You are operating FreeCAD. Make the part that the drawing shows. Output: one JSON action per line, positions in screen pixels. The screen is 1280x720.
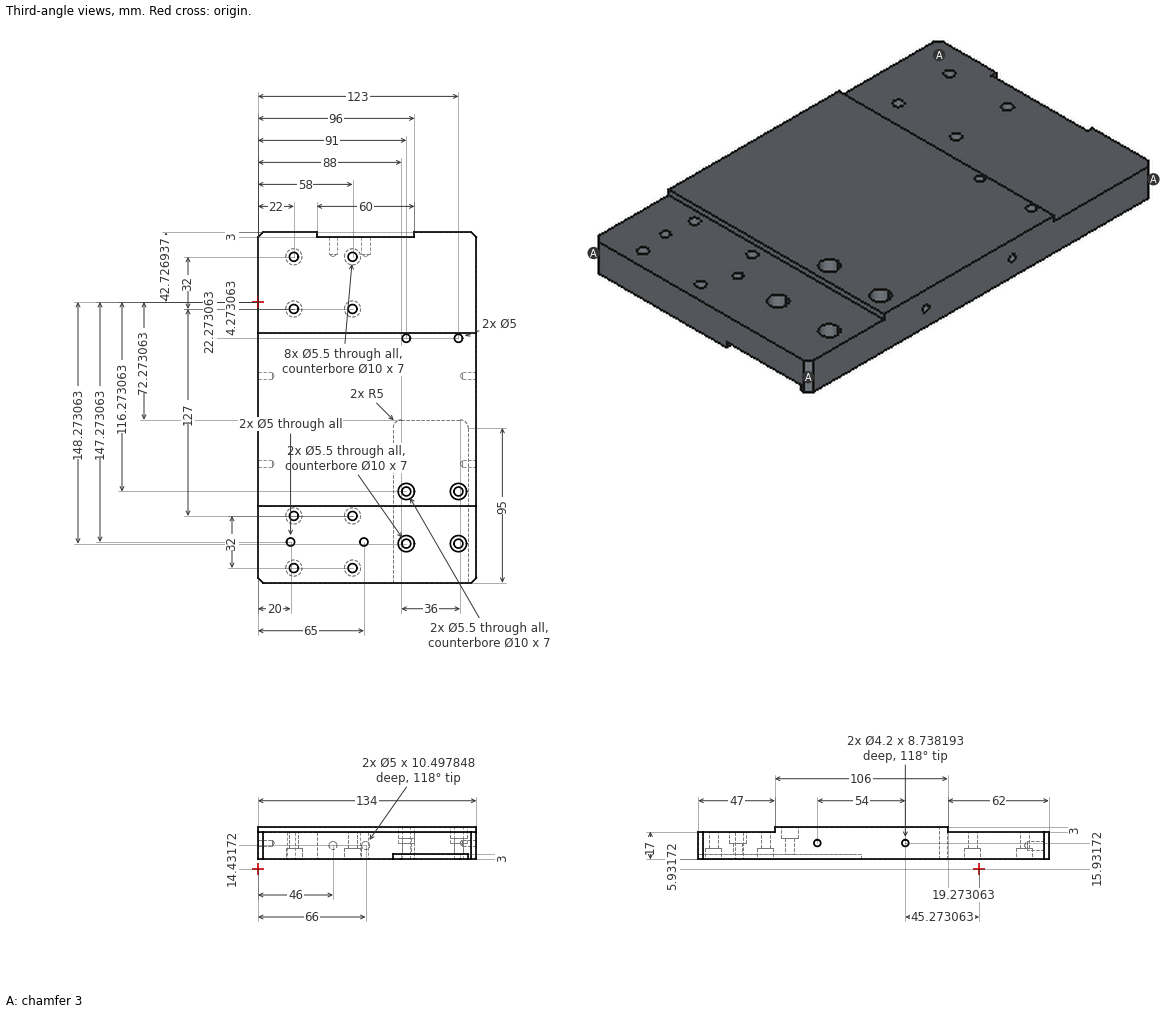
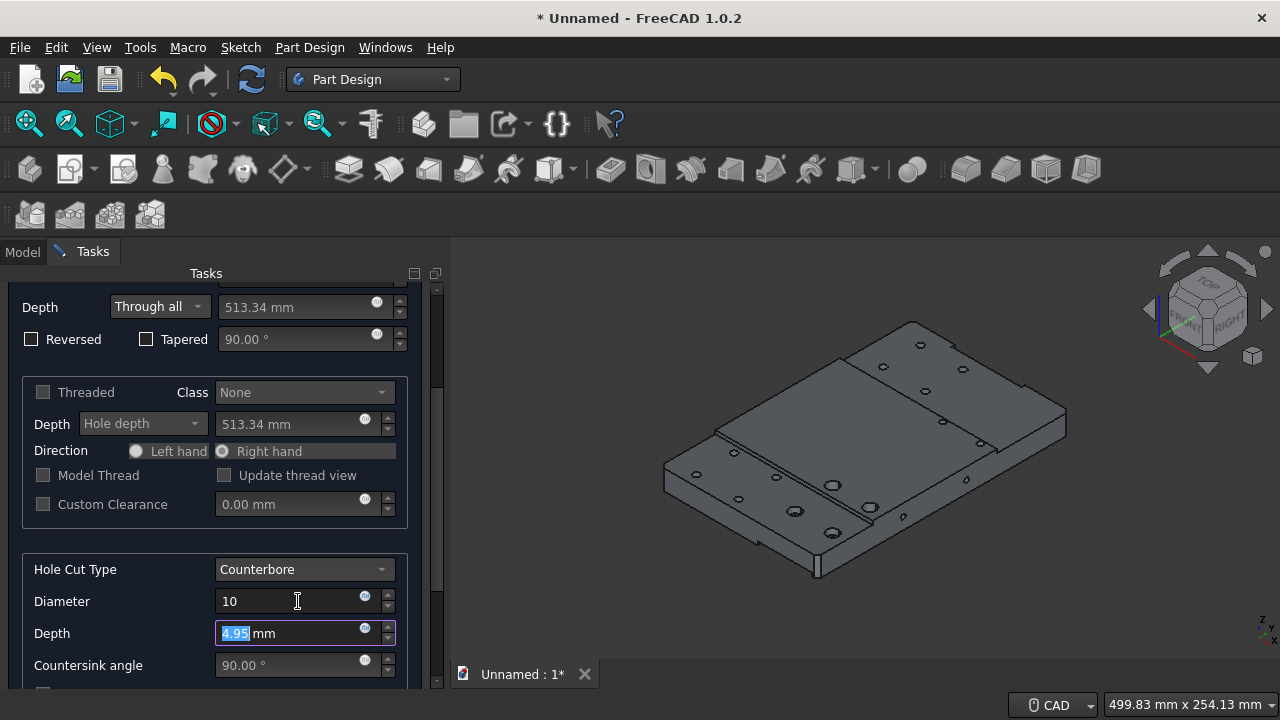
{"action": "type", "text": "7"}
{"action": "key", "text": "Tab"}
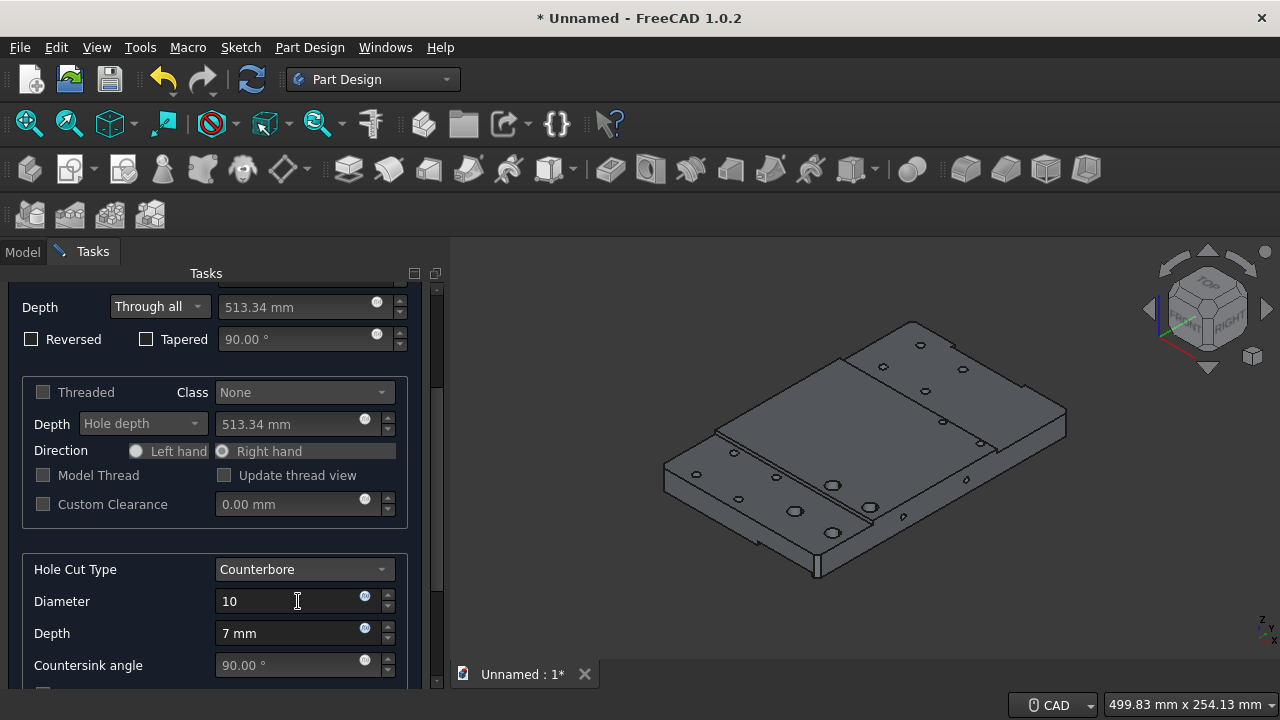
{"action": "scroll", "coordinate": [437, 486], "scroll_direction": "up", "scroll_amount": 4}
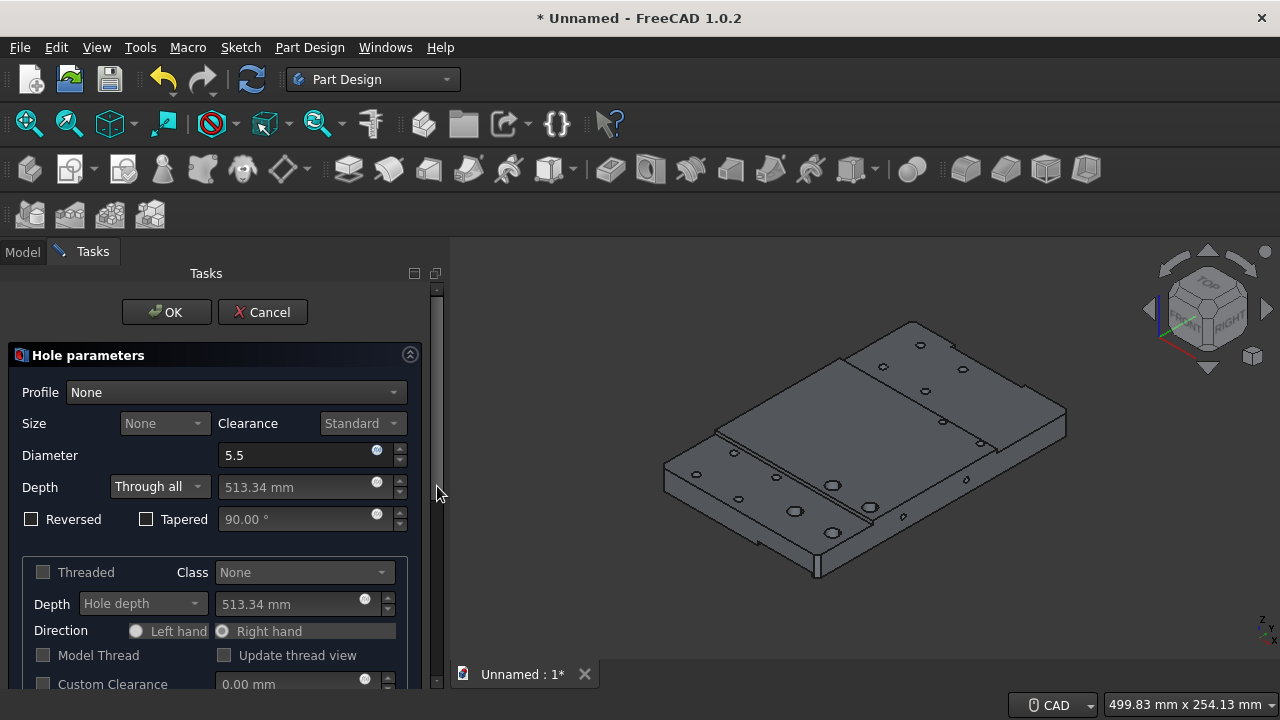
{"action": "left_click", "coordinate": [167, 312]}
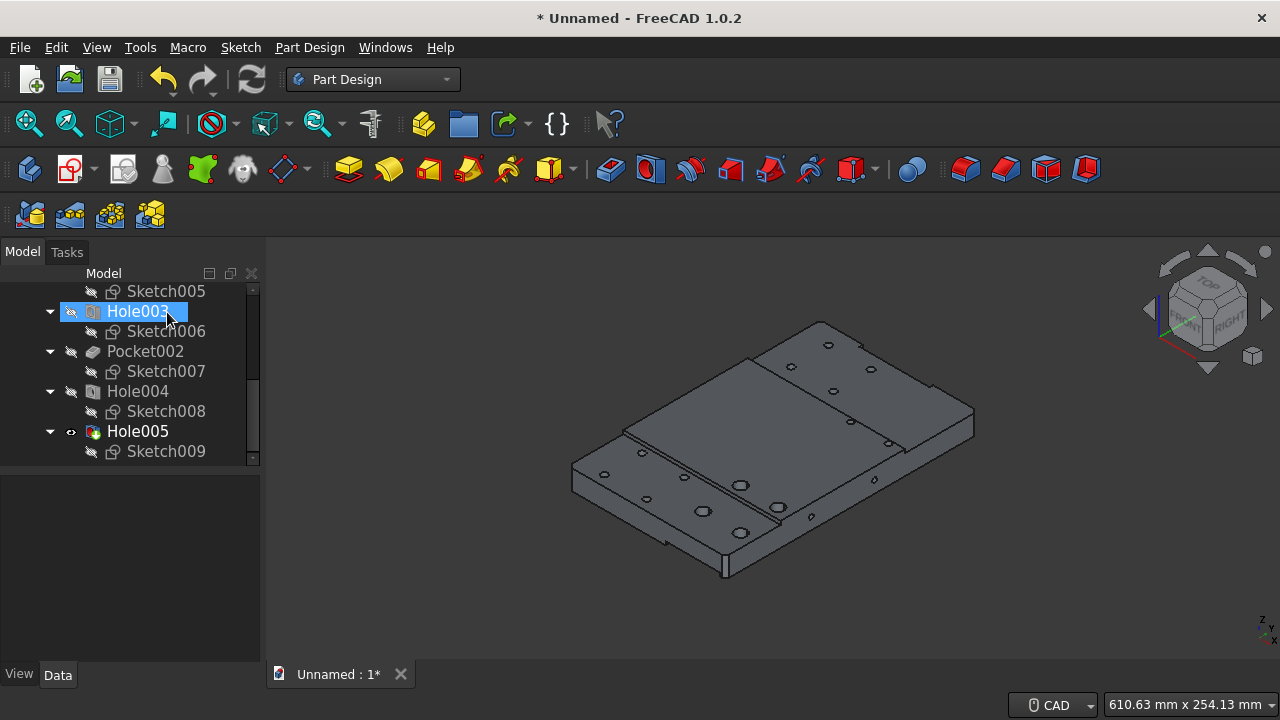
{"action": "left_click", "coordinate": [908, 412]}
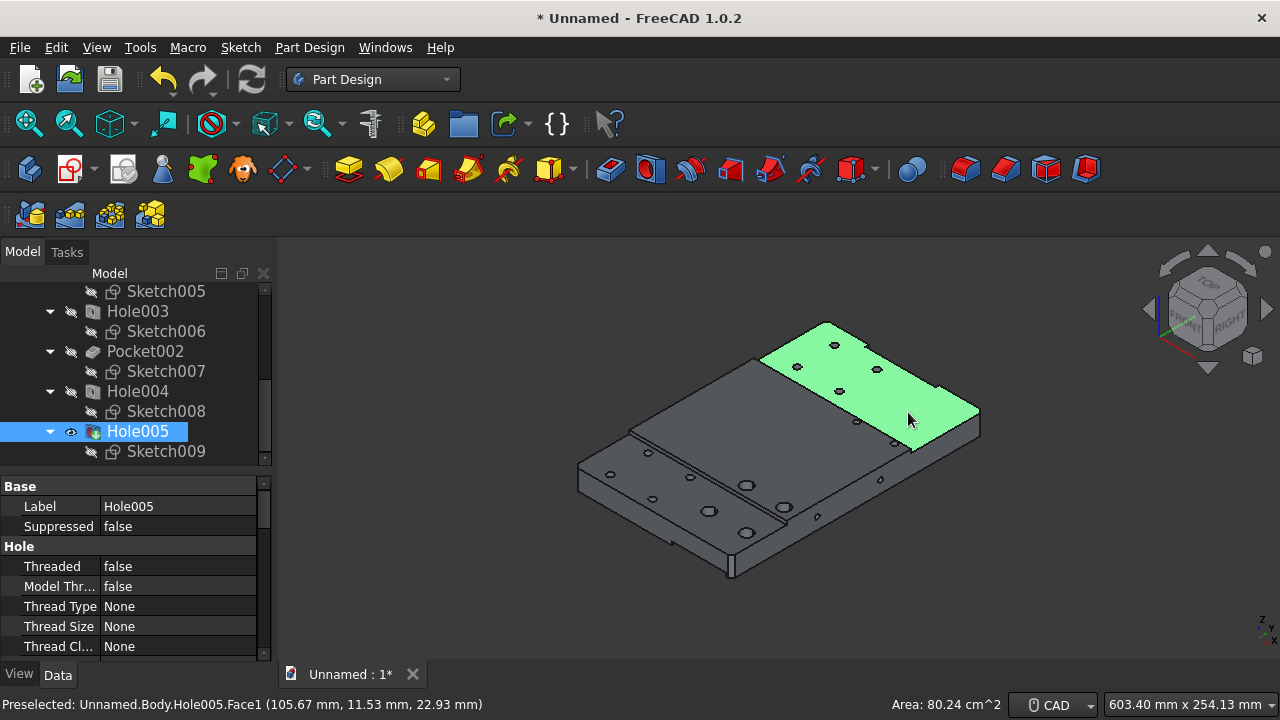
{"action": "left_click", "coordinate": [70, 170]}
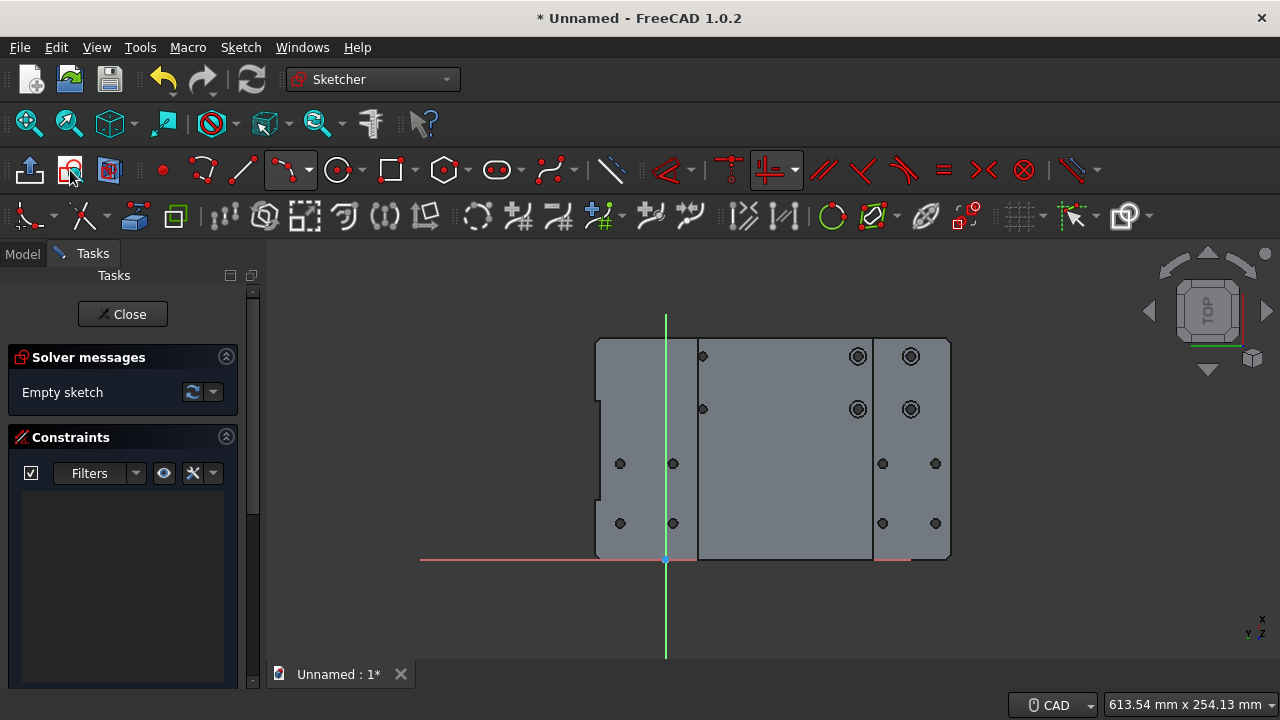
{"action": "scroll", "coordinate": [998, 507], "scroll_direction": "up", "scroll_amount": 6}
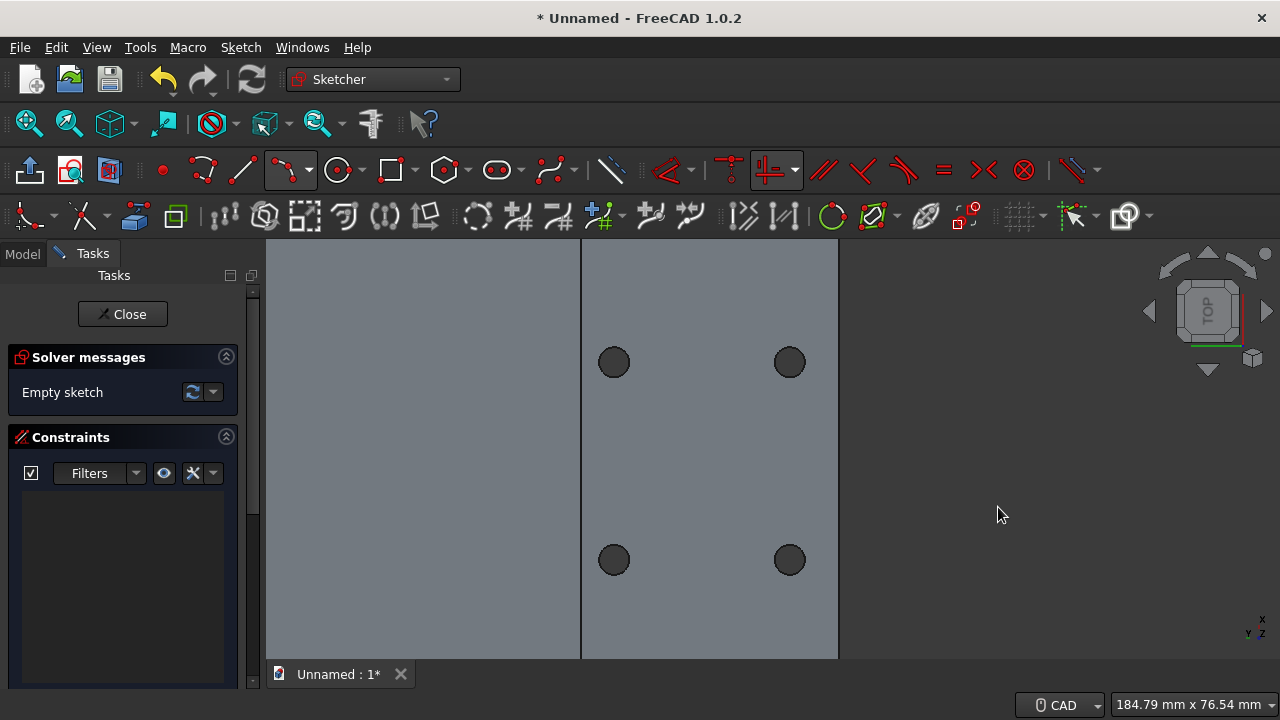
{"action": "left_click", "coordinate": [338, 170]}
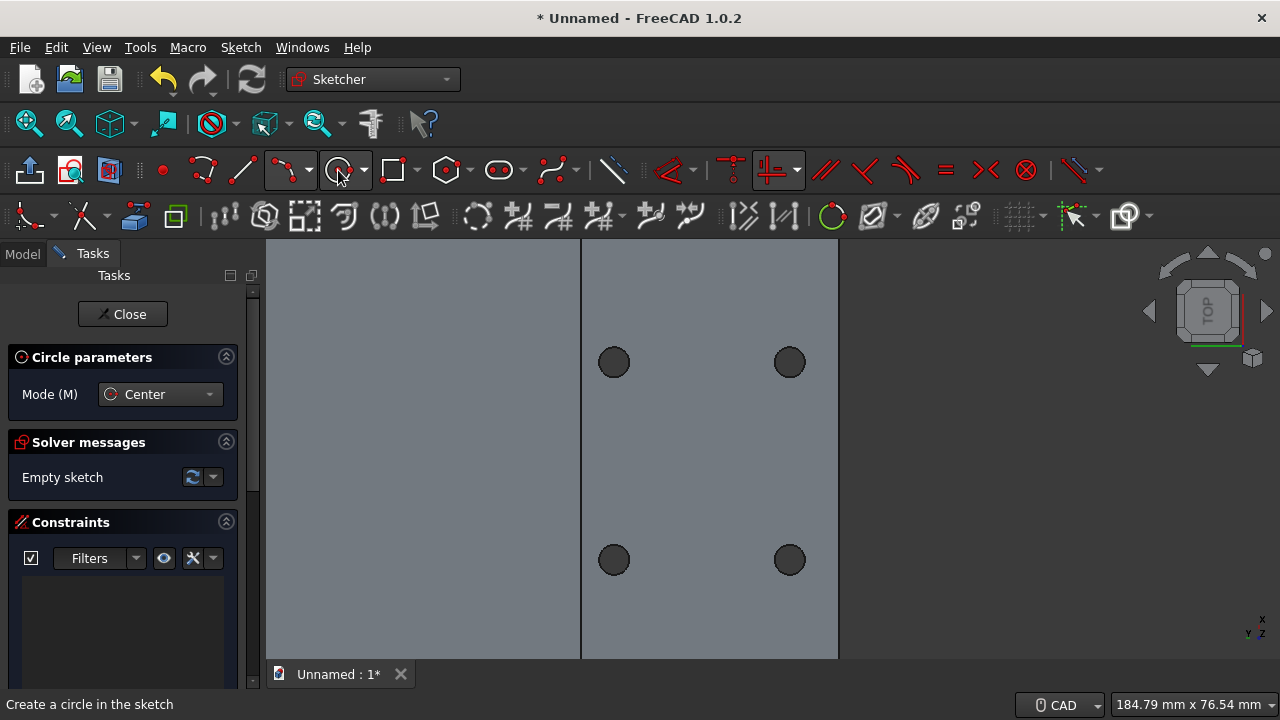
{"action": "scroll", "coordinate": [702, 571], "scroll_direction": "up", "scroll_amount": 3}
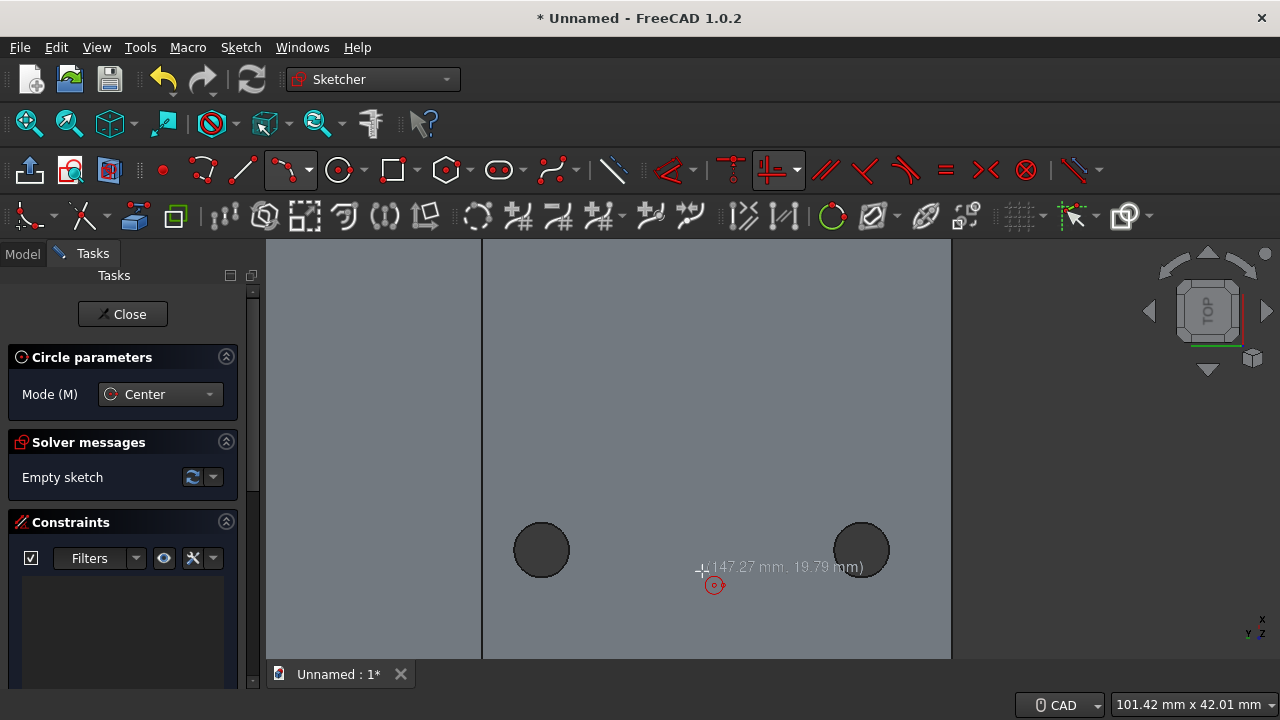
{"action": "left_click", "coordinate": [702, 570]}
{"action": "mouse_move", "coordinate": [719, 552]}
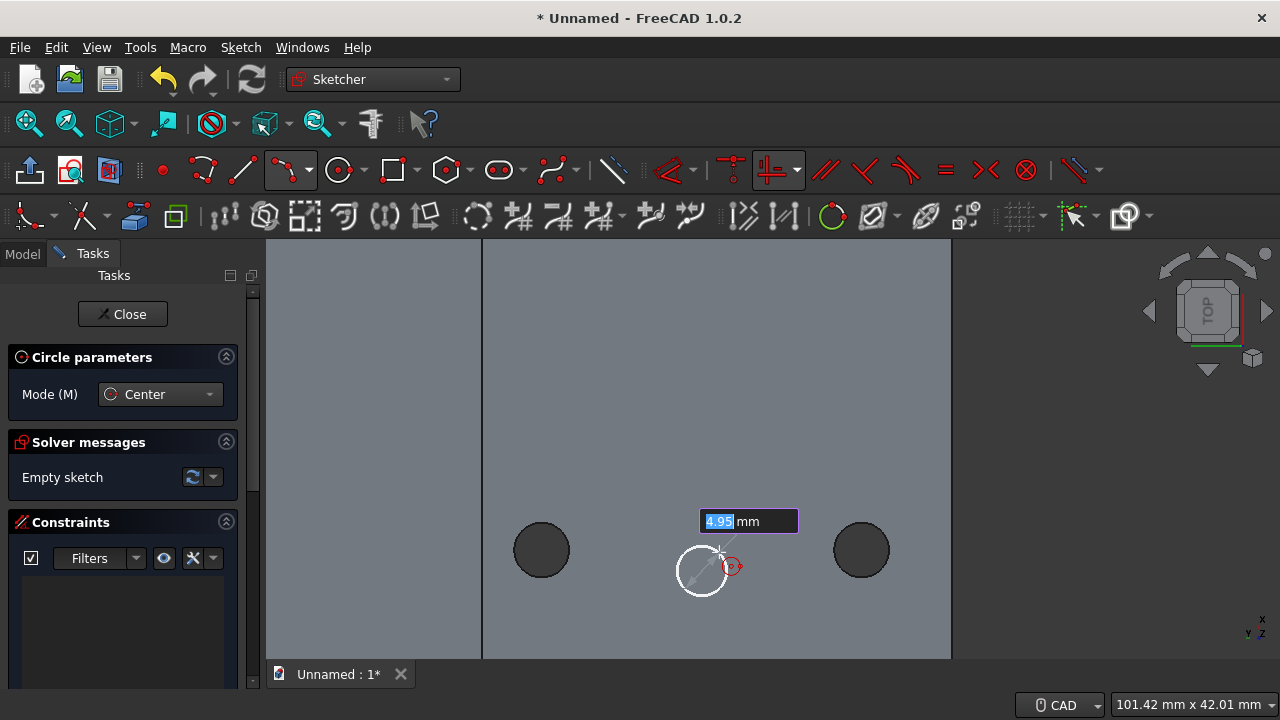
{"action": "type", "text": "5"}
{"action": "key", "text": "Return"}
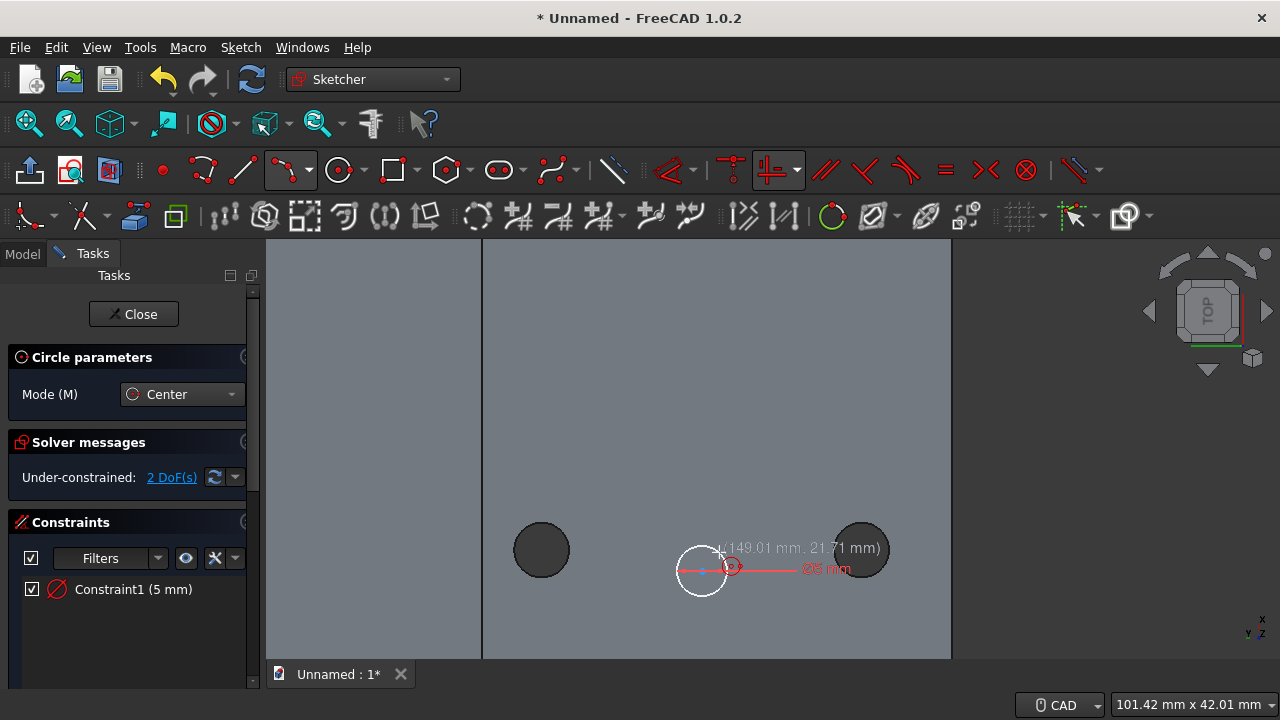
{"action": "scroll", "coordinate": [708, 575], "scroll_direction": "down", "scroll_amount": 3}